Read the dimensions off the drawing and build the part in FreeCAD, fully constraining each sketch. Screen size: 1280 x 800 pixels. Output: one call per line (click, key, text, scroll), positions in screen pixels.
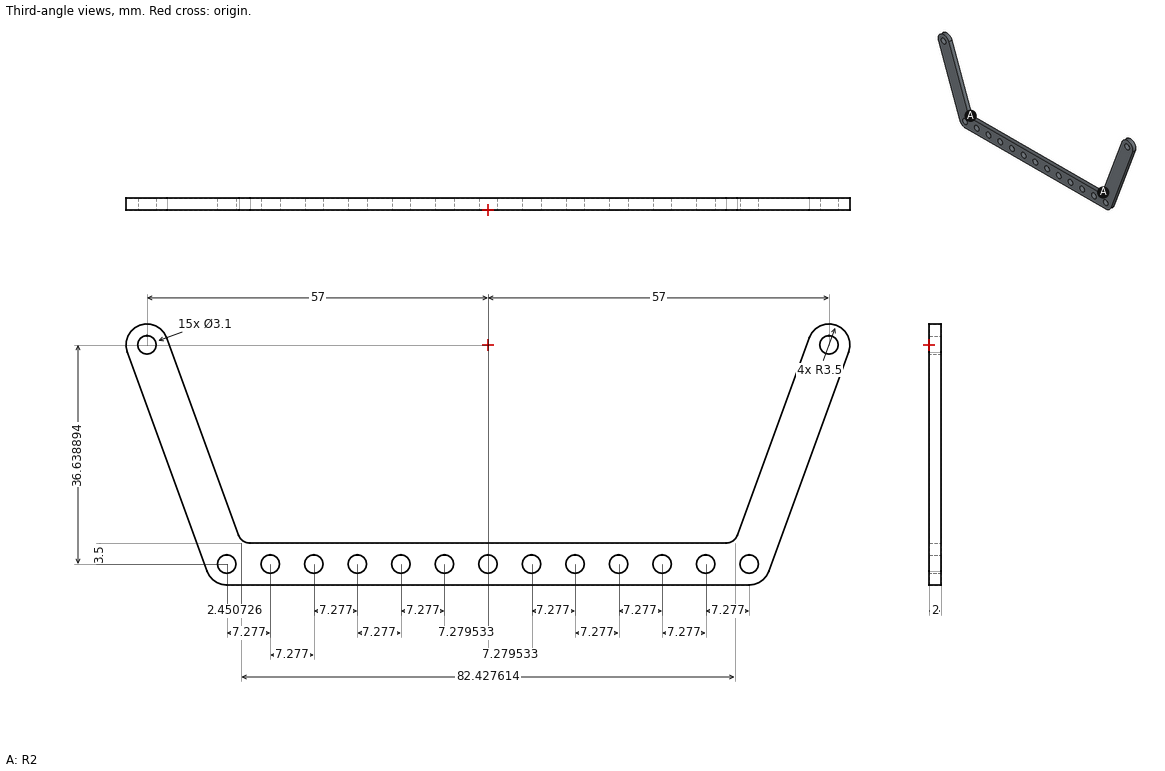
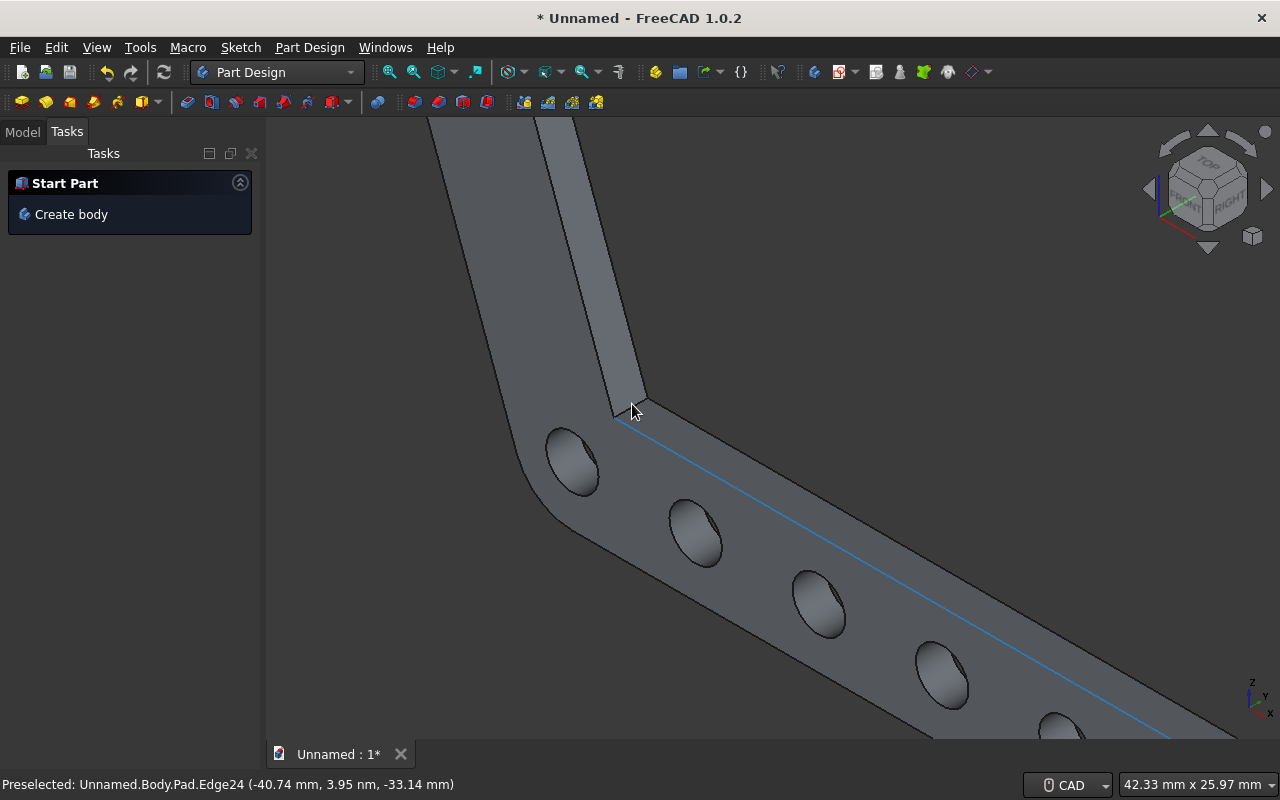
key(v)
key(f)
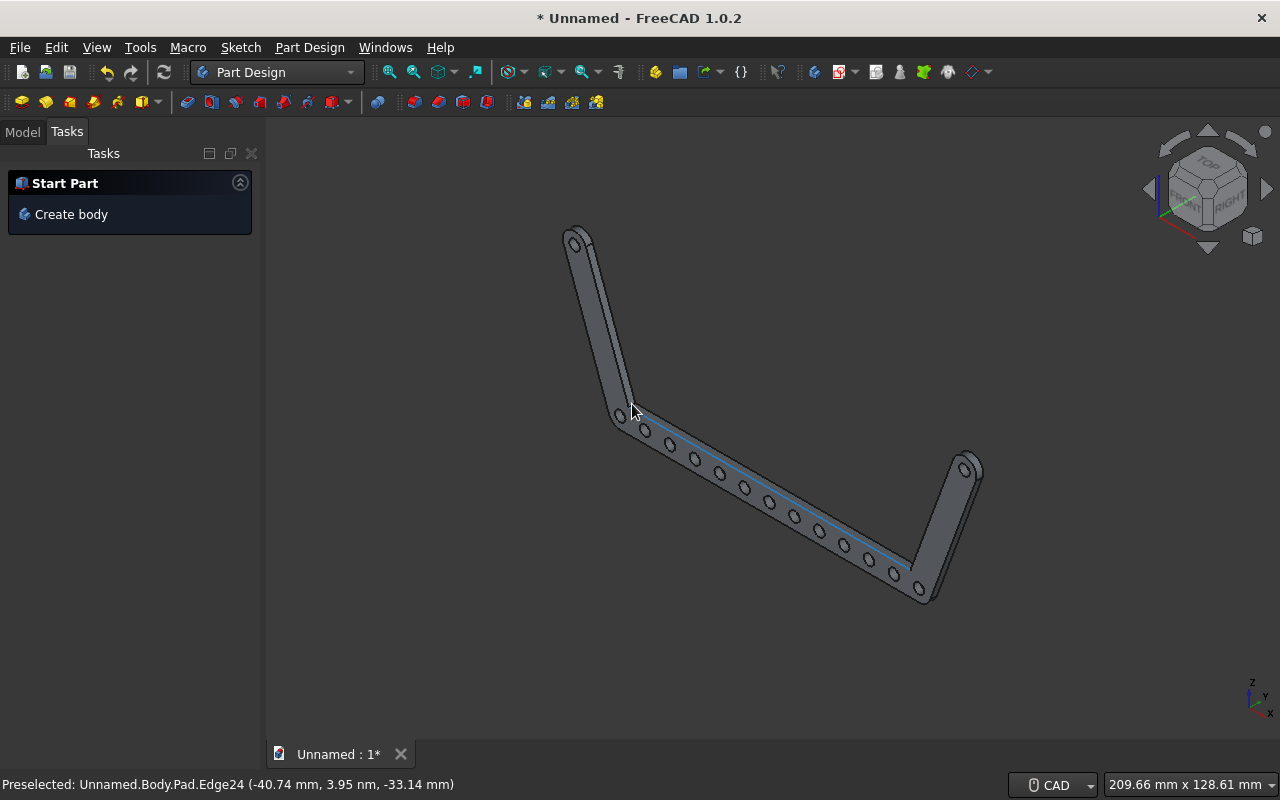
key(2)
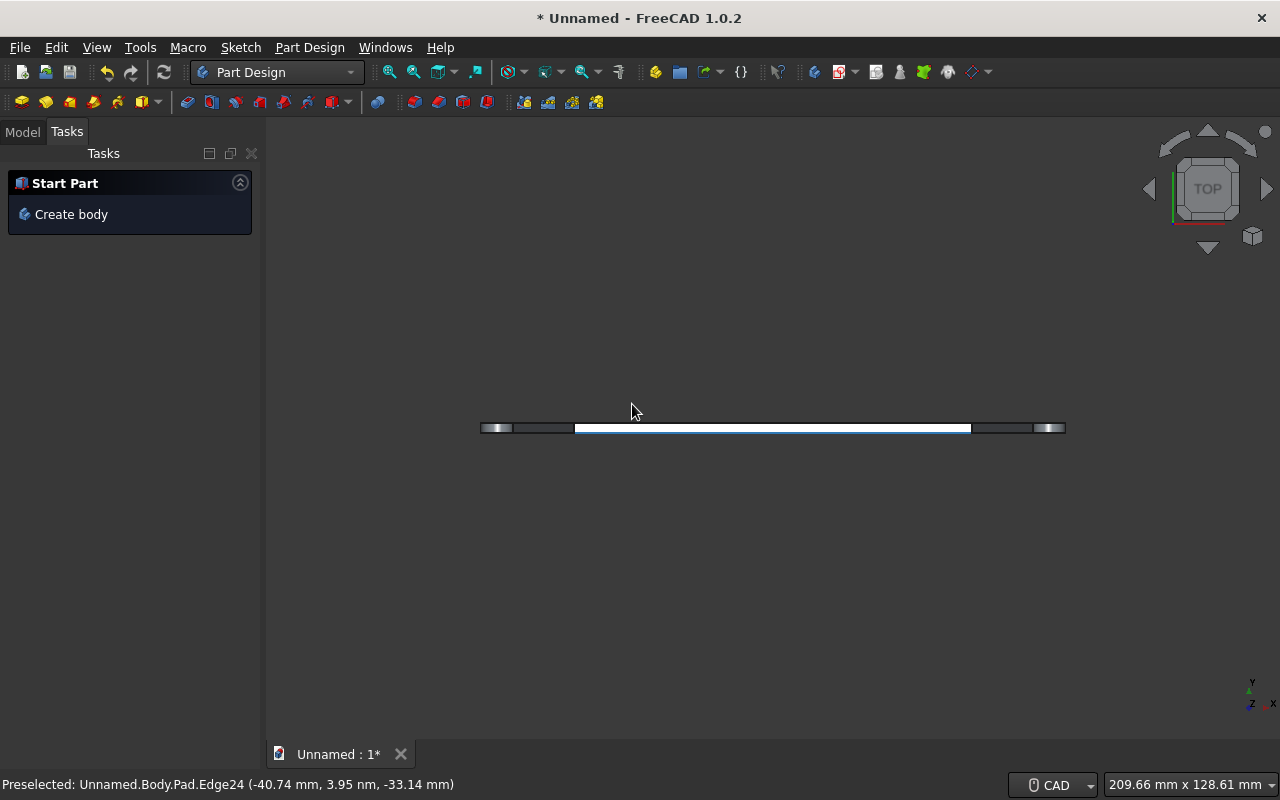
scroll(574, 427, up, 8)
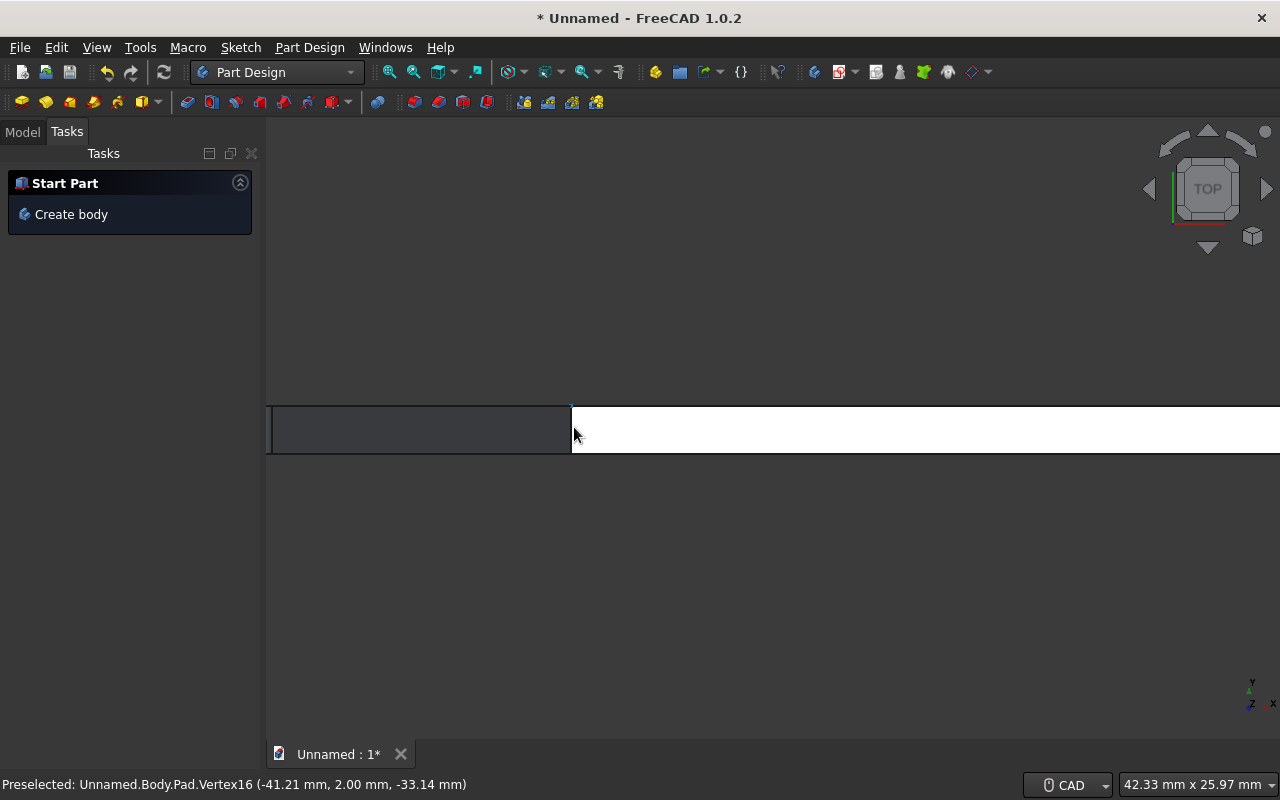
key(v)
key(f)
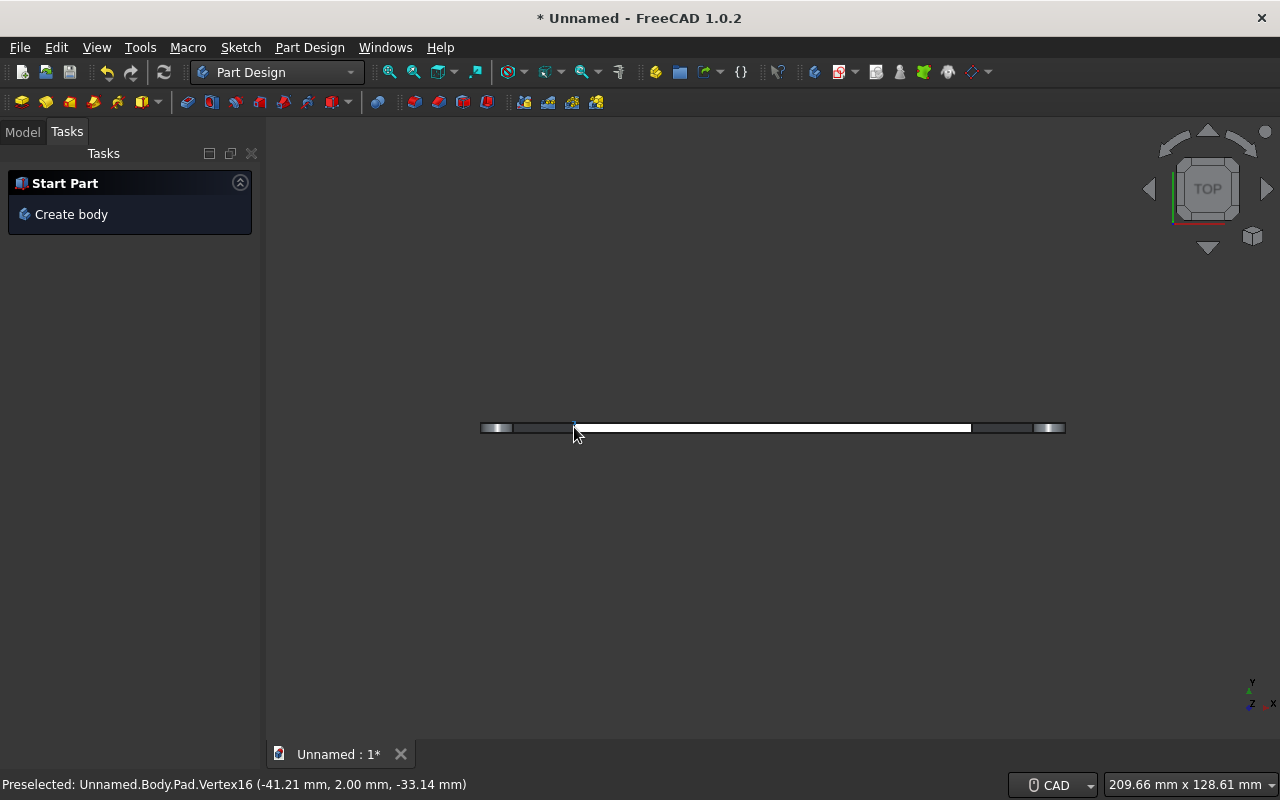
key(1)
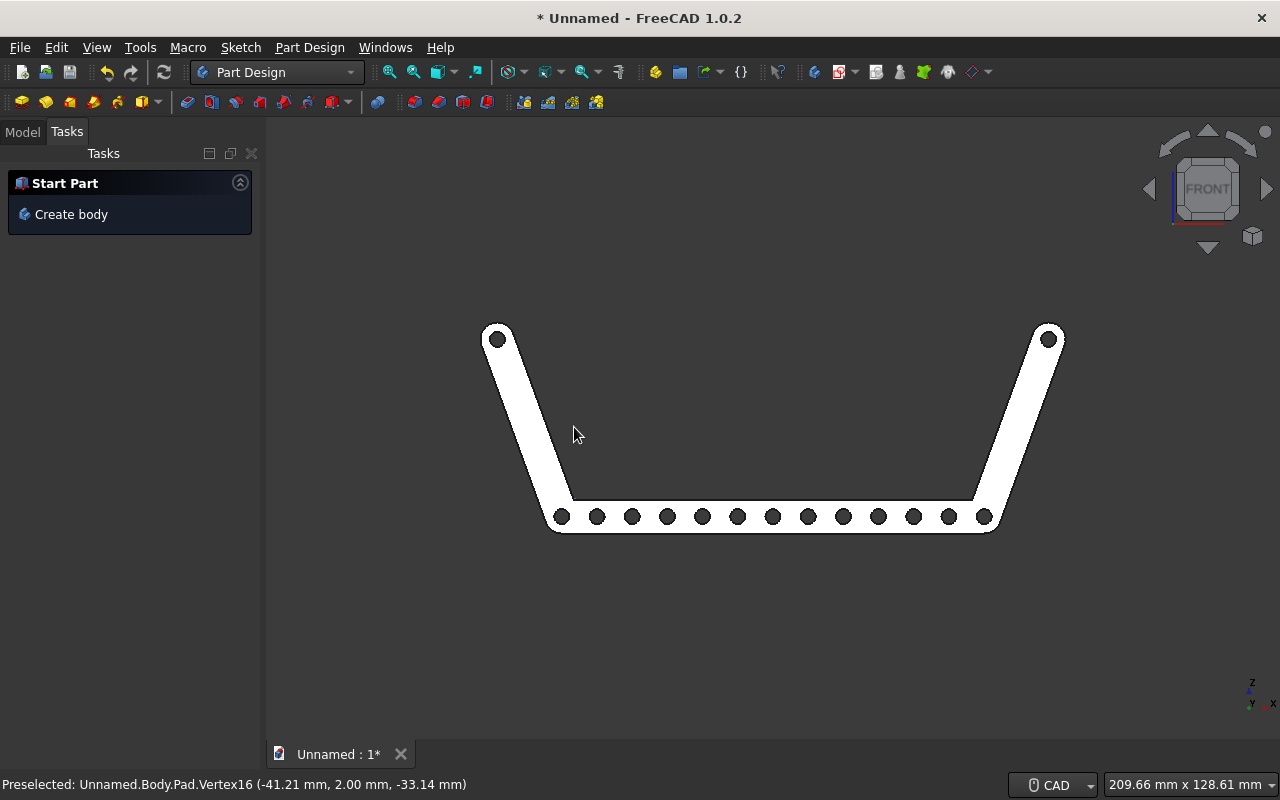
scroll(574, 499, up, 8)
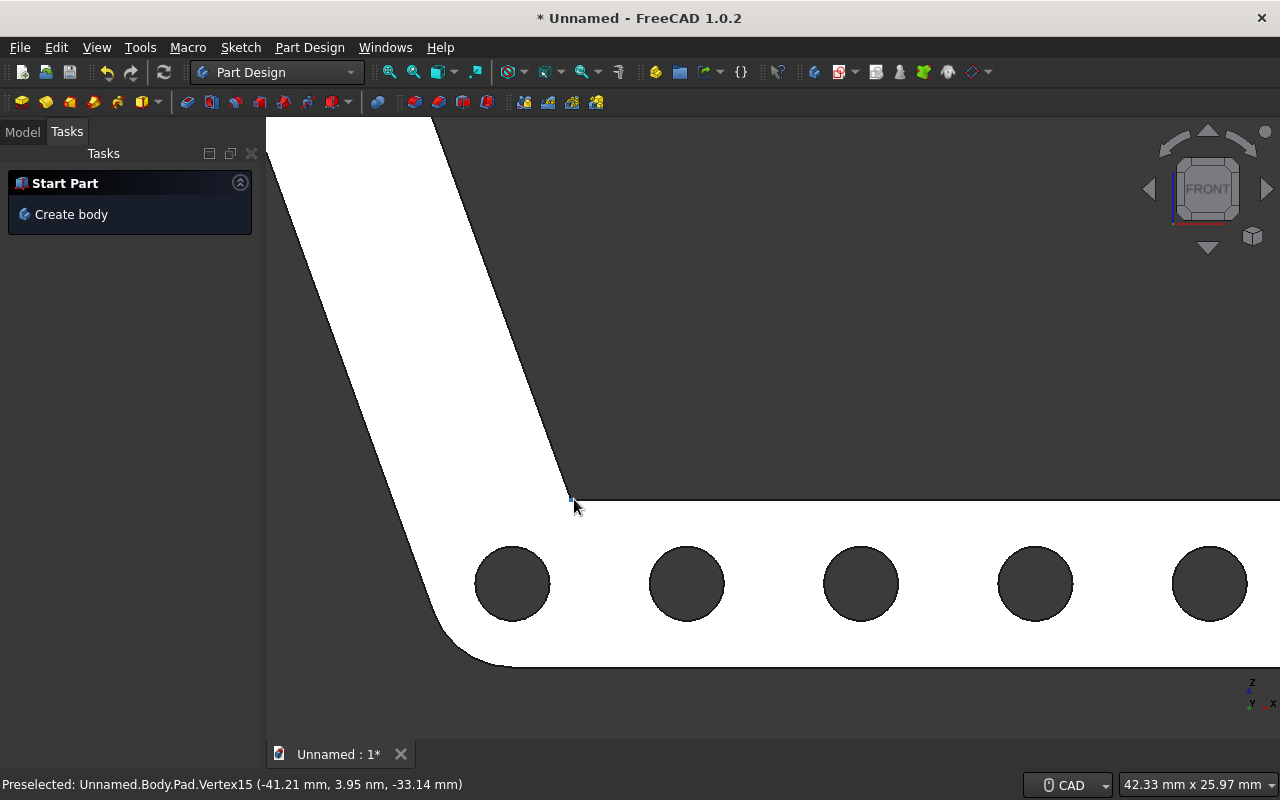
key(v)
key(f)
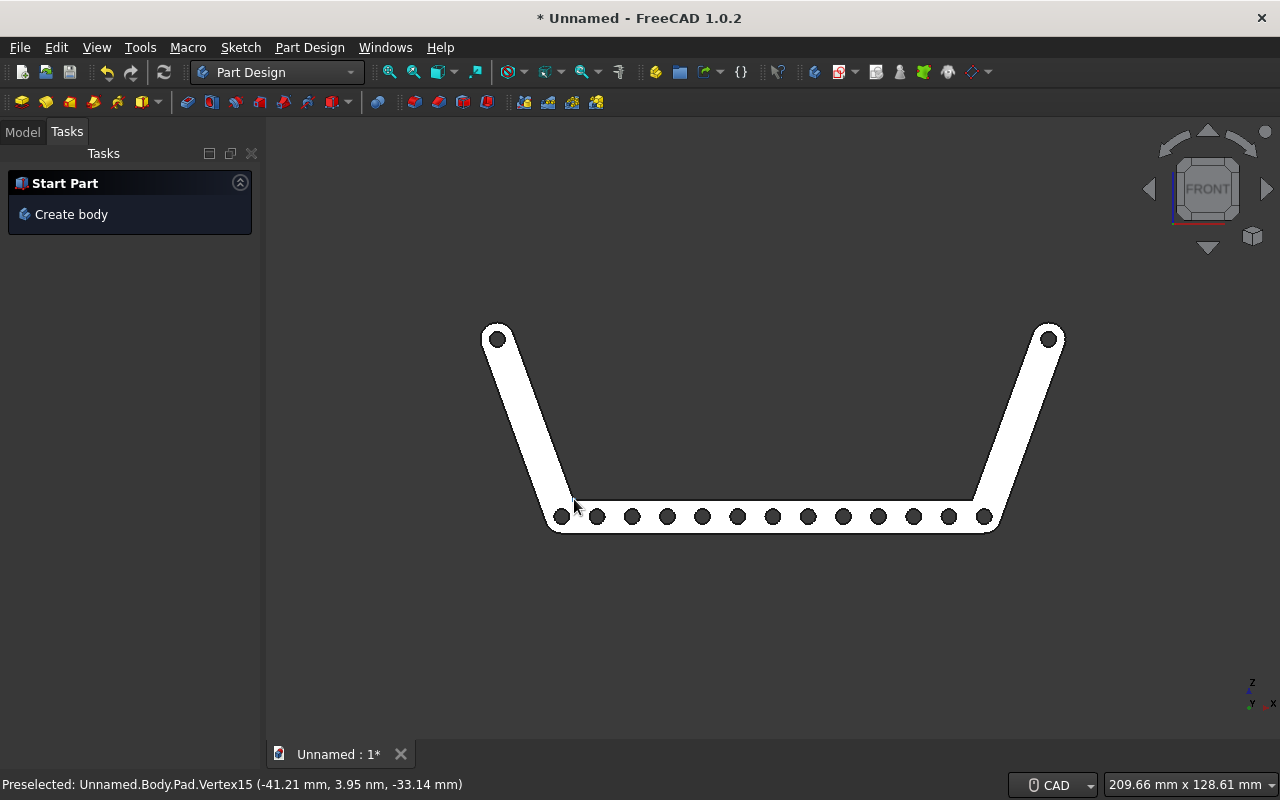
key(3)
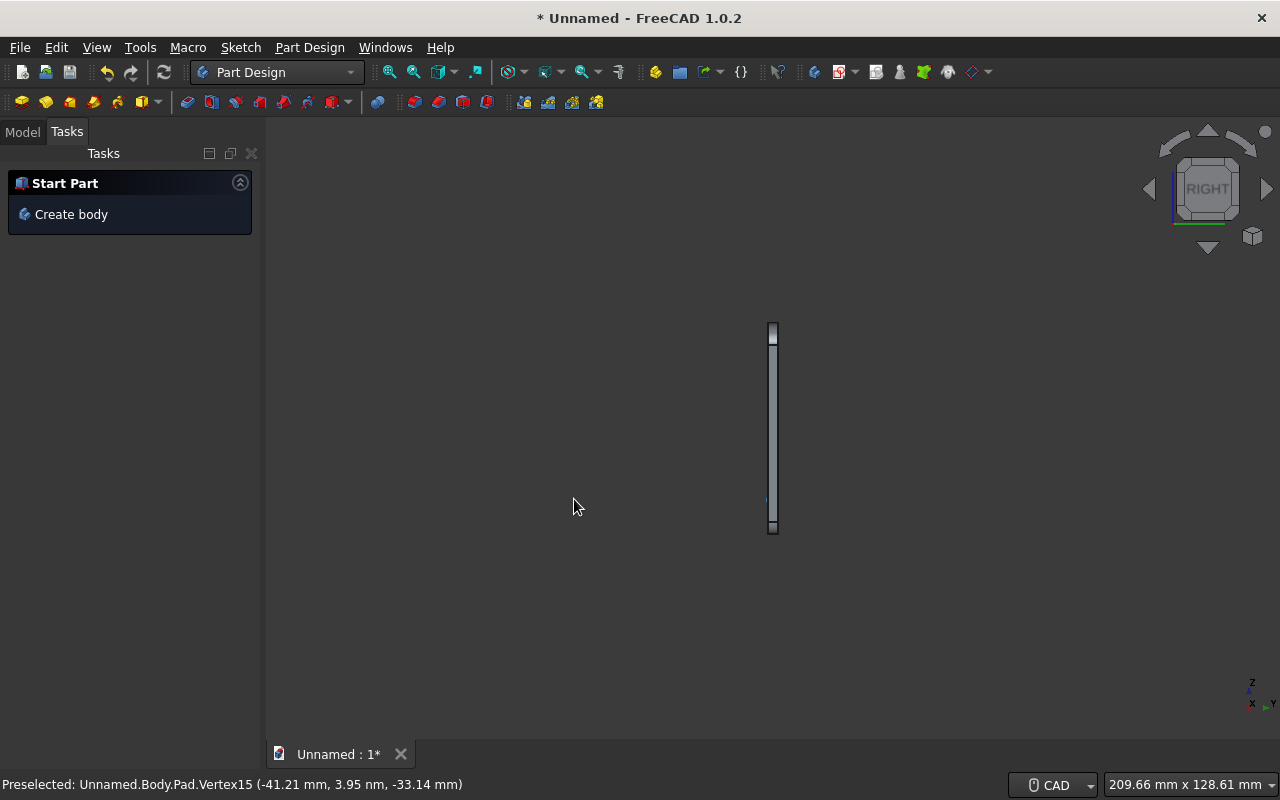
key(v)
key(f)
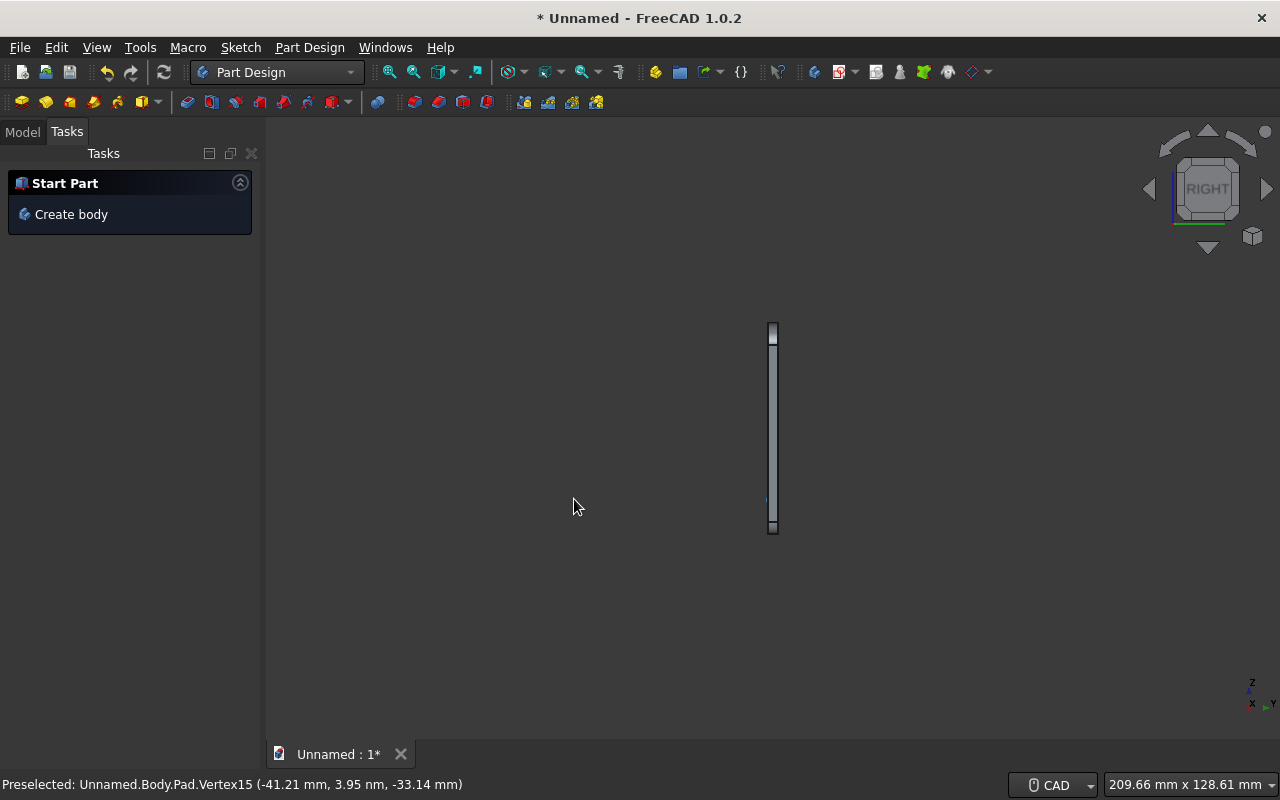
scroll(773, 499, up, 8)